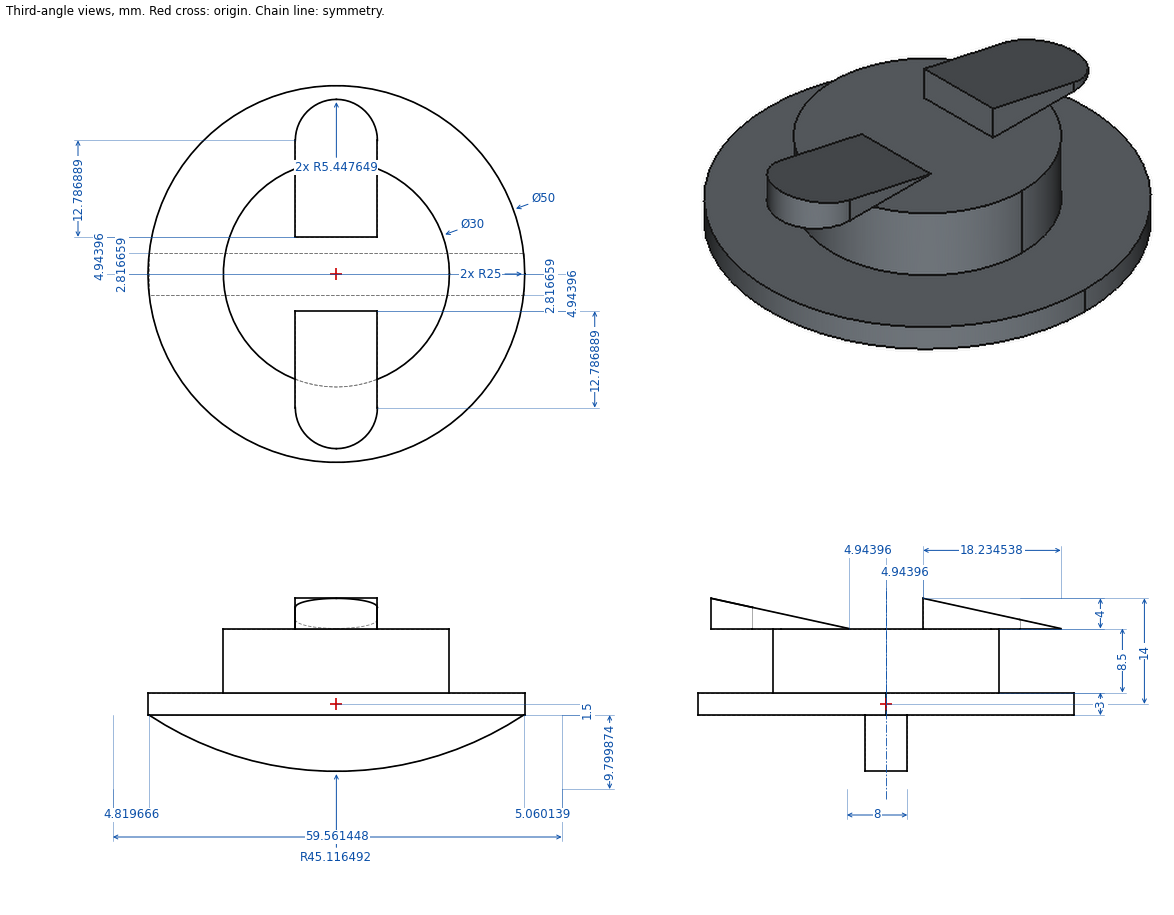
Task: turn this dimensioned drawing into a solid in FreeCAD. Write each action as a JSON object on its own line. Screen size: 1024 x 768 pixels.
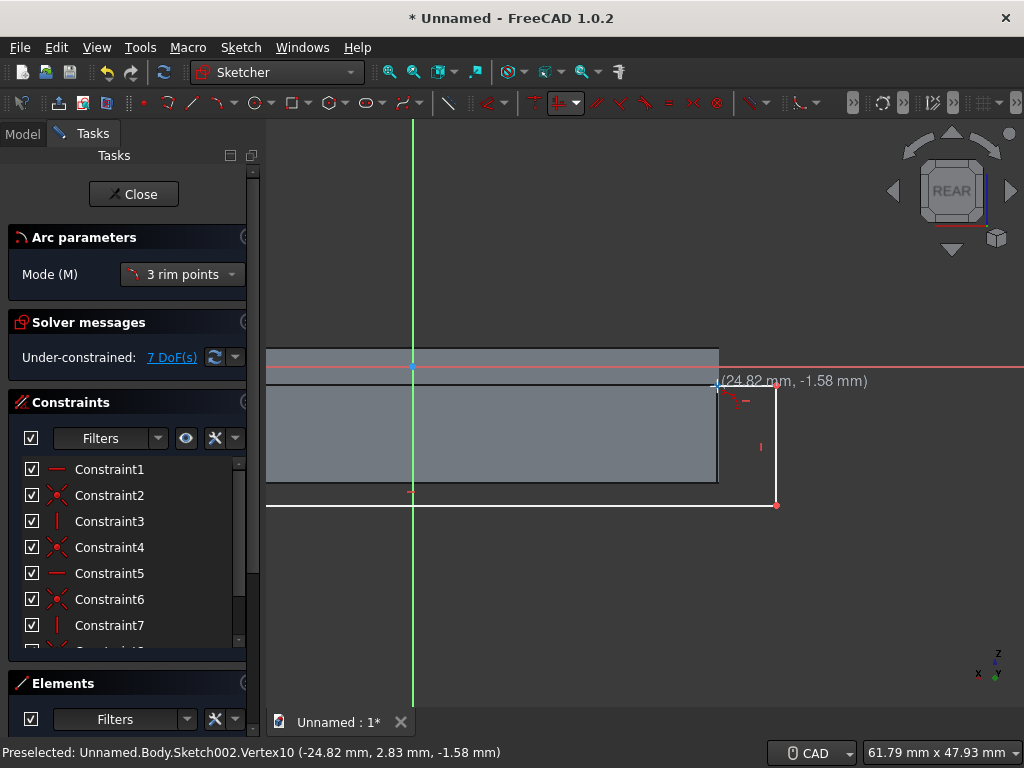
{"action": "scroll", "coordinate": [778, 385], "scroll_direction": "down", "scroll_amount": 3}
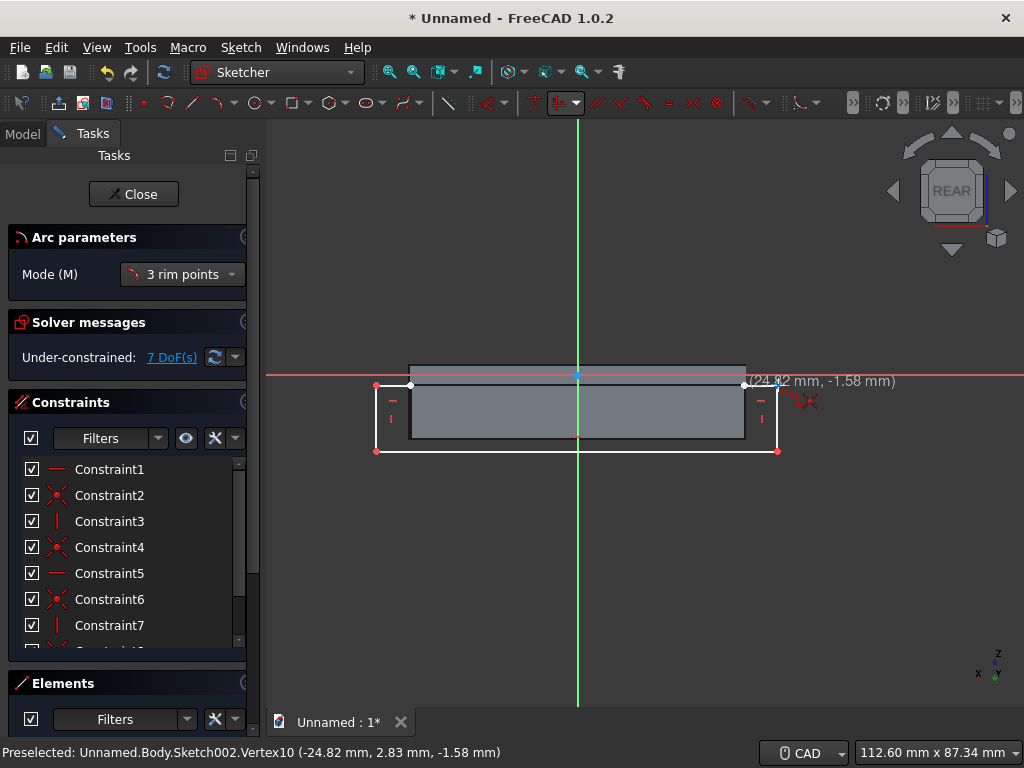
{"action": "scroll", "coordinate": [411, 385], "scroll_direction": "up", "scroll_amount": 3}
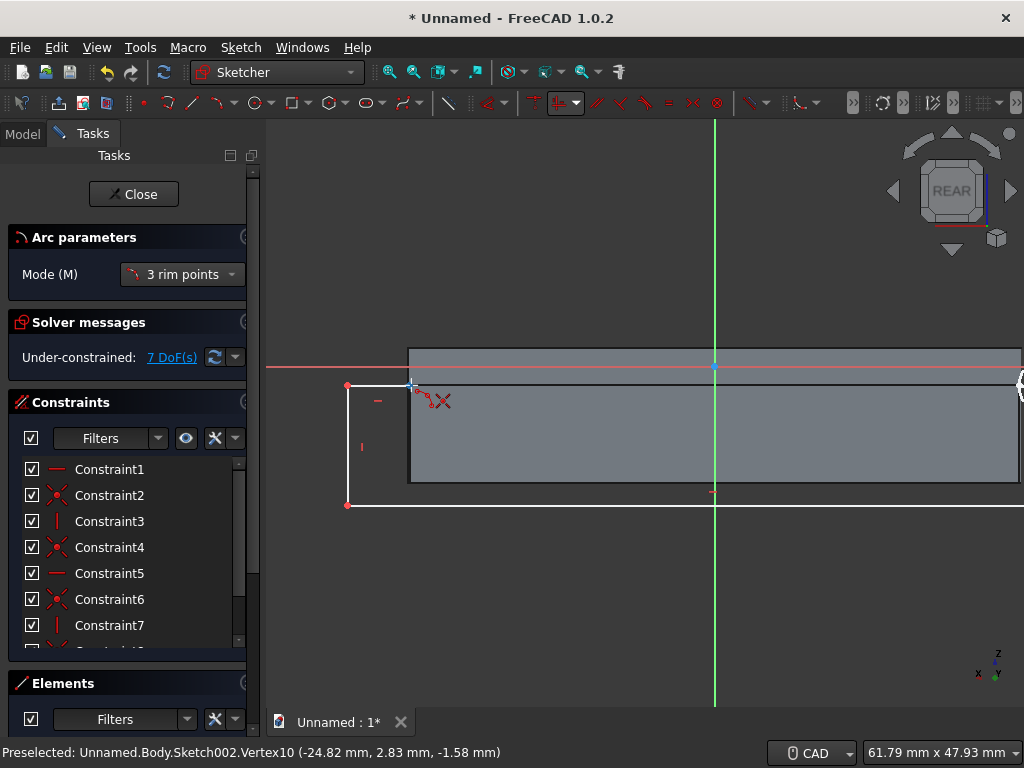
{"action": "left_click", "coordinate": [410, 386]}
{"action": "left_click", "coordinate": [650, 473]}
{"action": "key", "text": "Escape"}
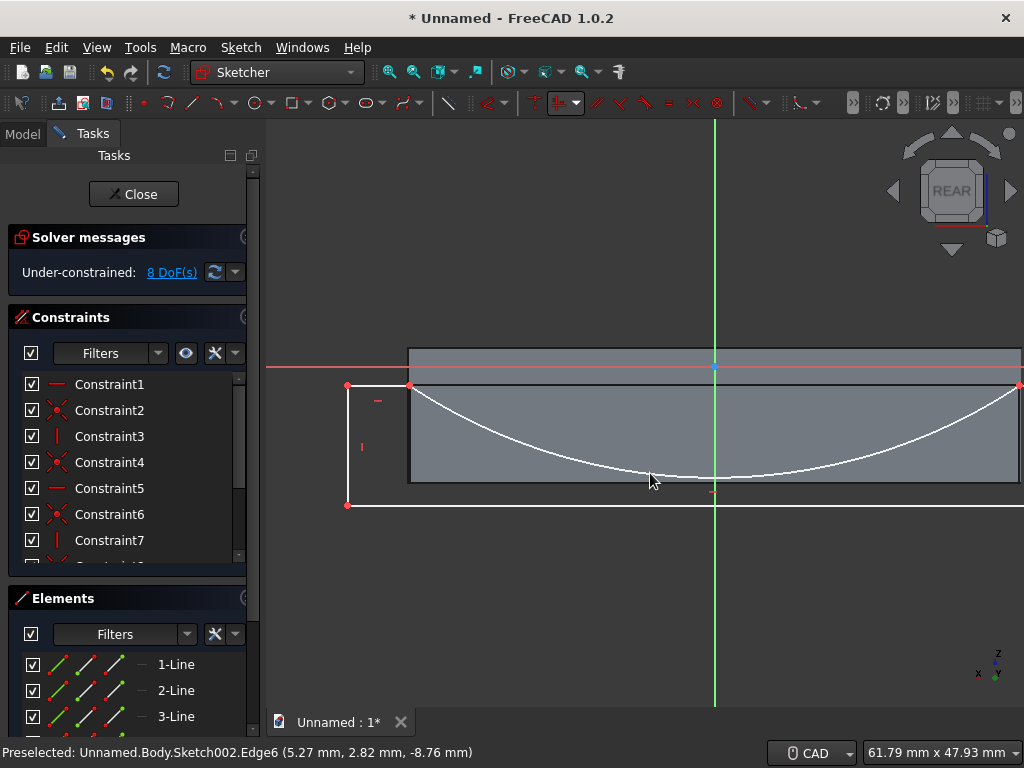
{"action": "scroll", "coordinate": [410, 385], "scroll_direction": "down", "scroll_amount": 3}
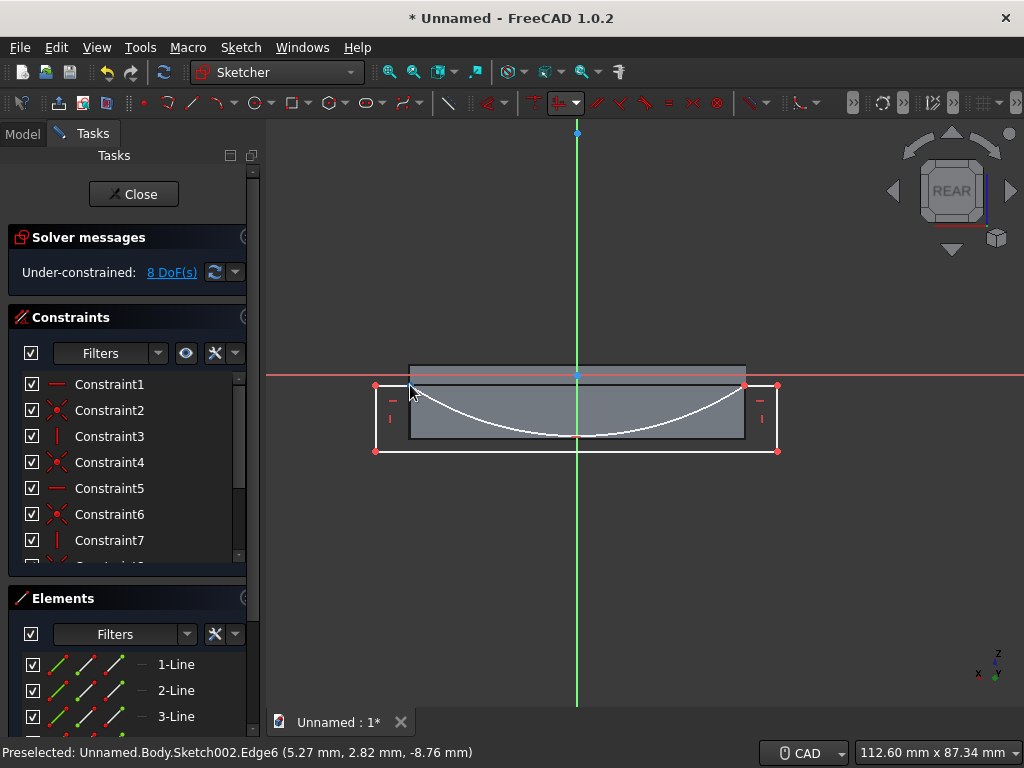
{"action": "scroll", "coordinate": [576, 679], "scroll_direction": "down", "scroll_amount": 1}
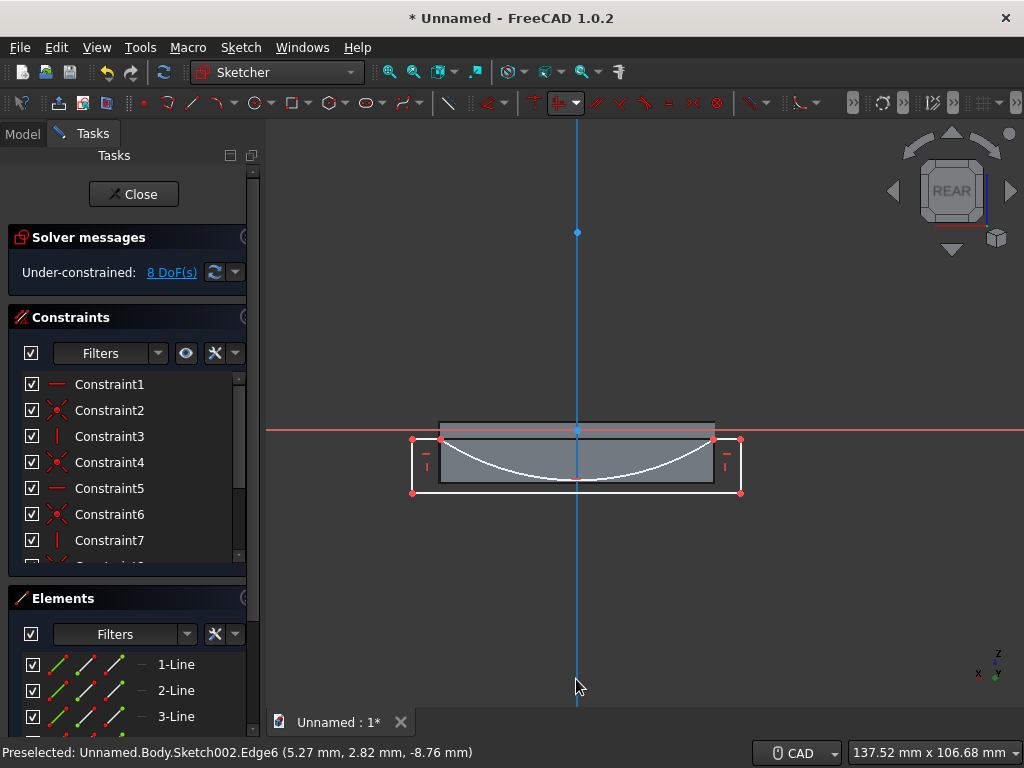
{"action": "left_click", "coordinate": [577, 233]}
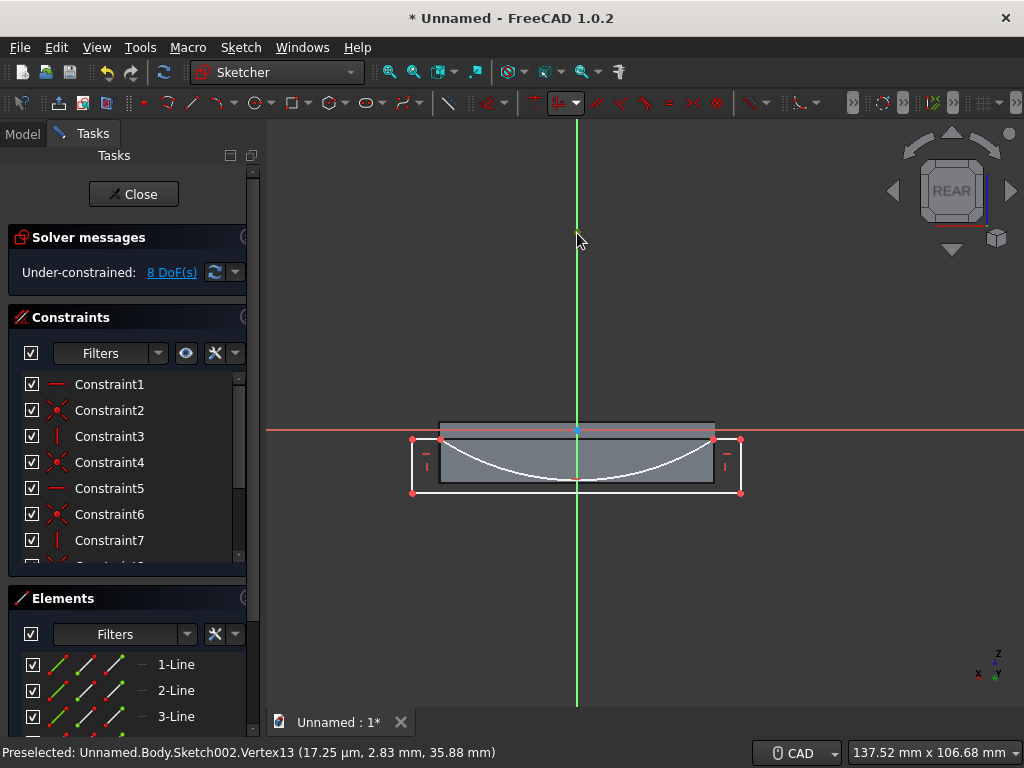
{"action": "left_click", "coordinate": [577, 641]}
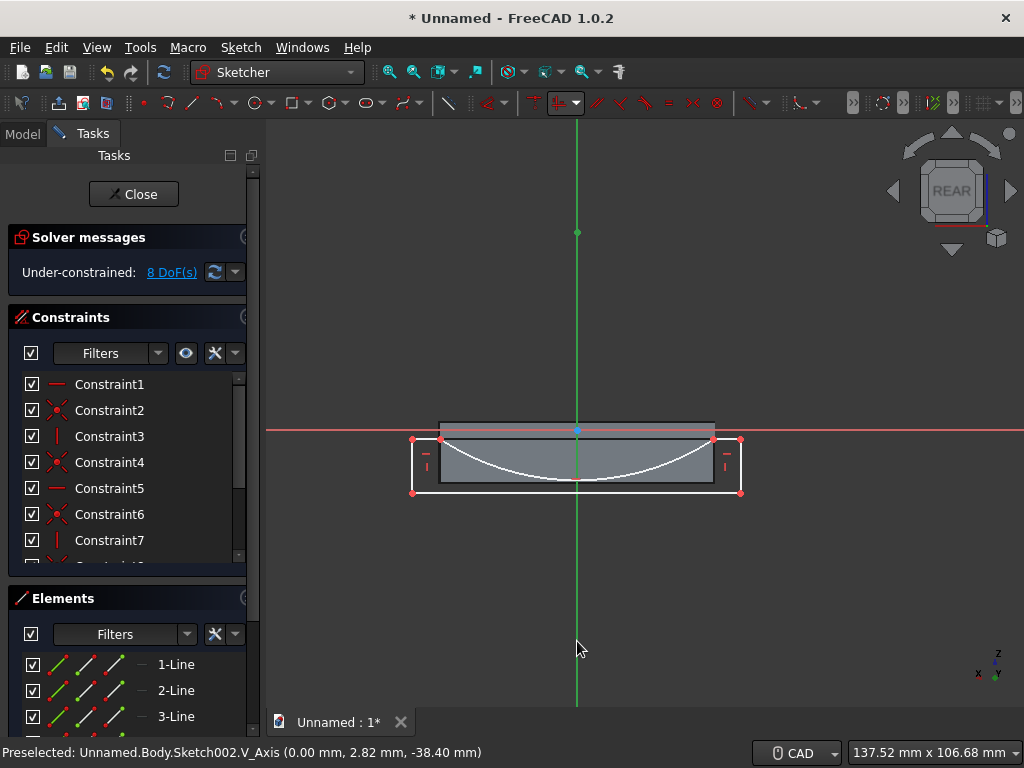
{"action": "left_click", "coordinate": [534, 104]}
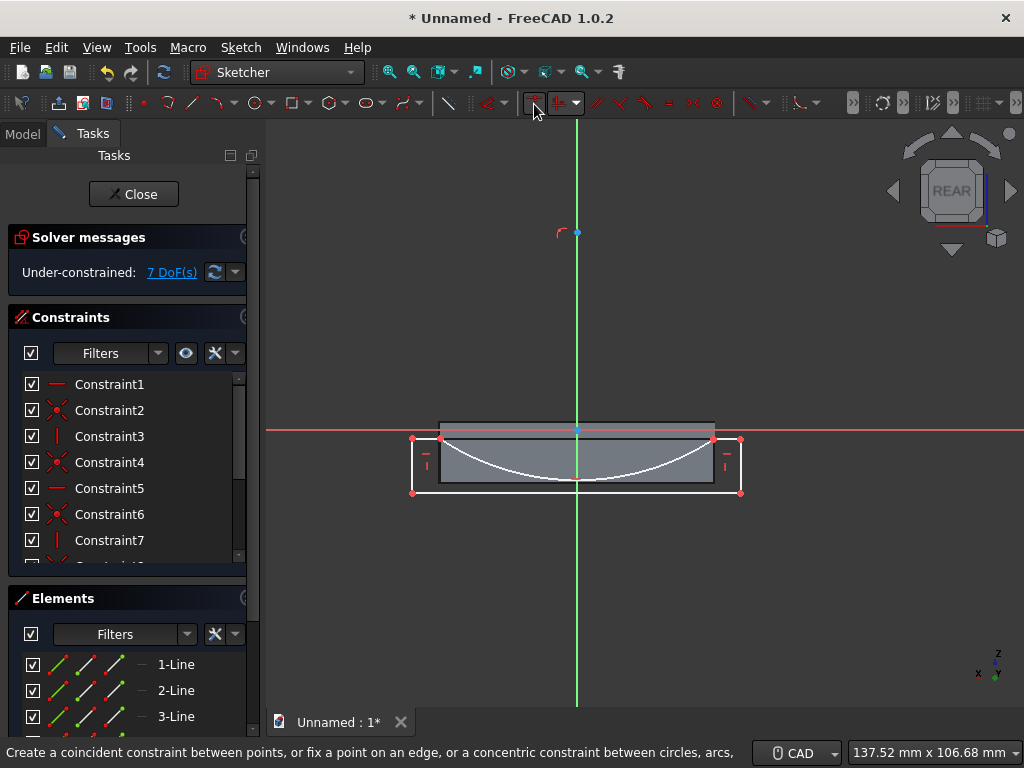
{"action": "left_click", "coordinate": [488, 104]}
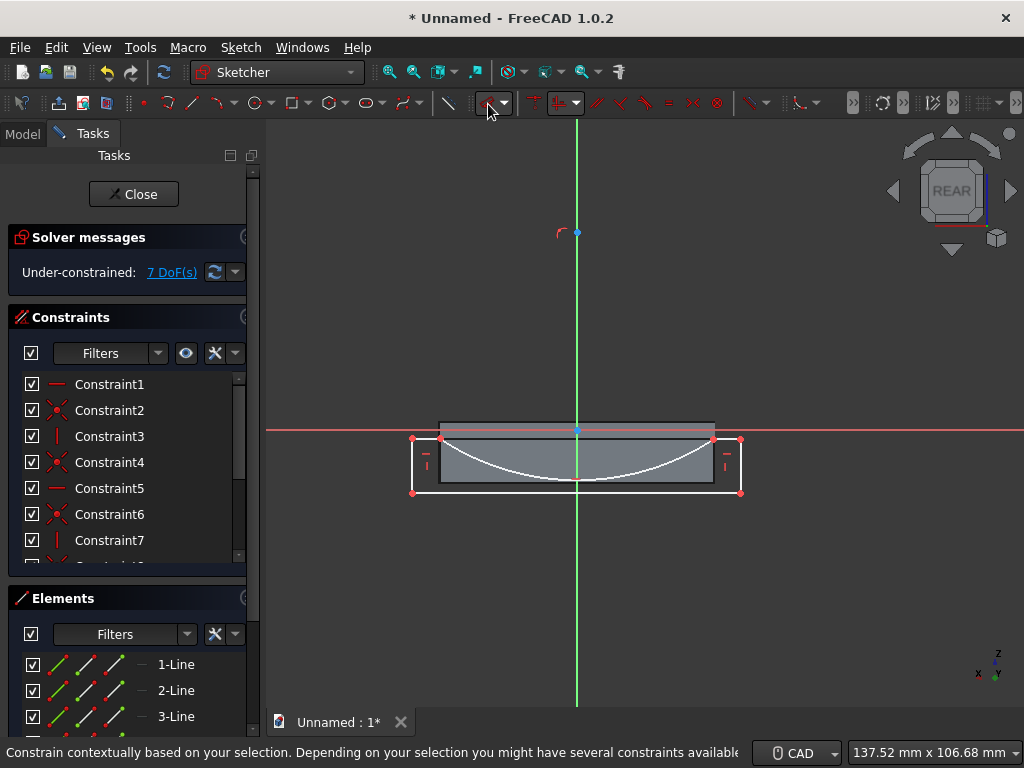
{"action": "left_click", "coordinate": [520, 473]}
{"action": "left_click", "coordinate": [314, 325]}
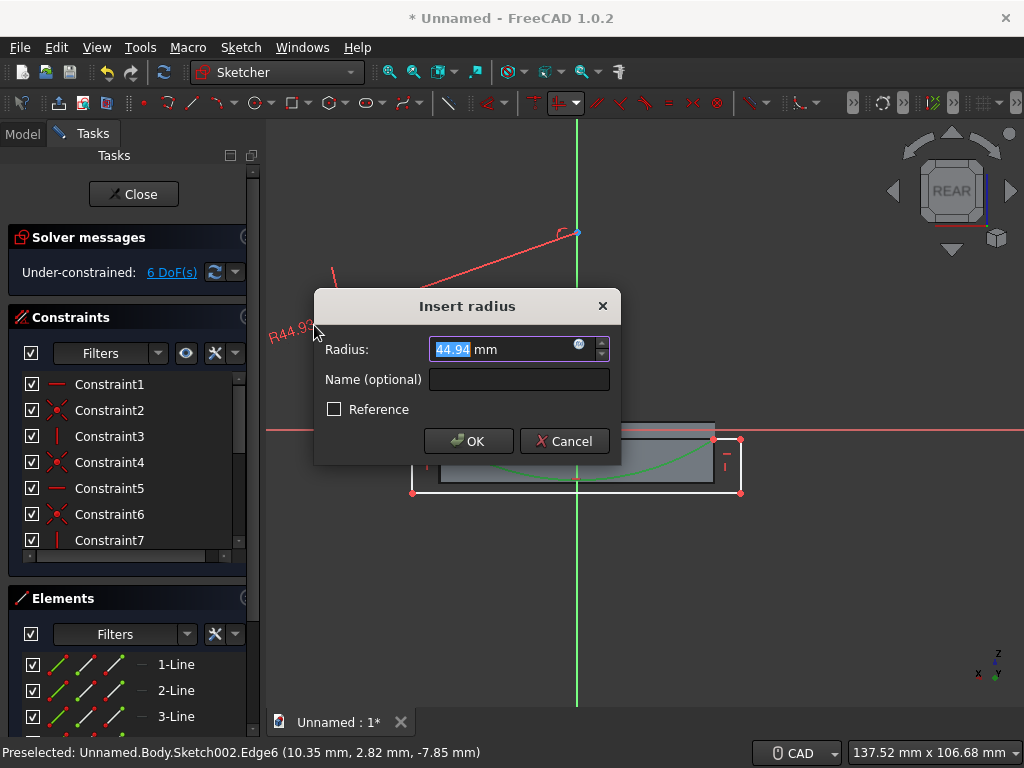
{"action": "type", "text": "45.116492"}
{"action": "key", "text": "Return"}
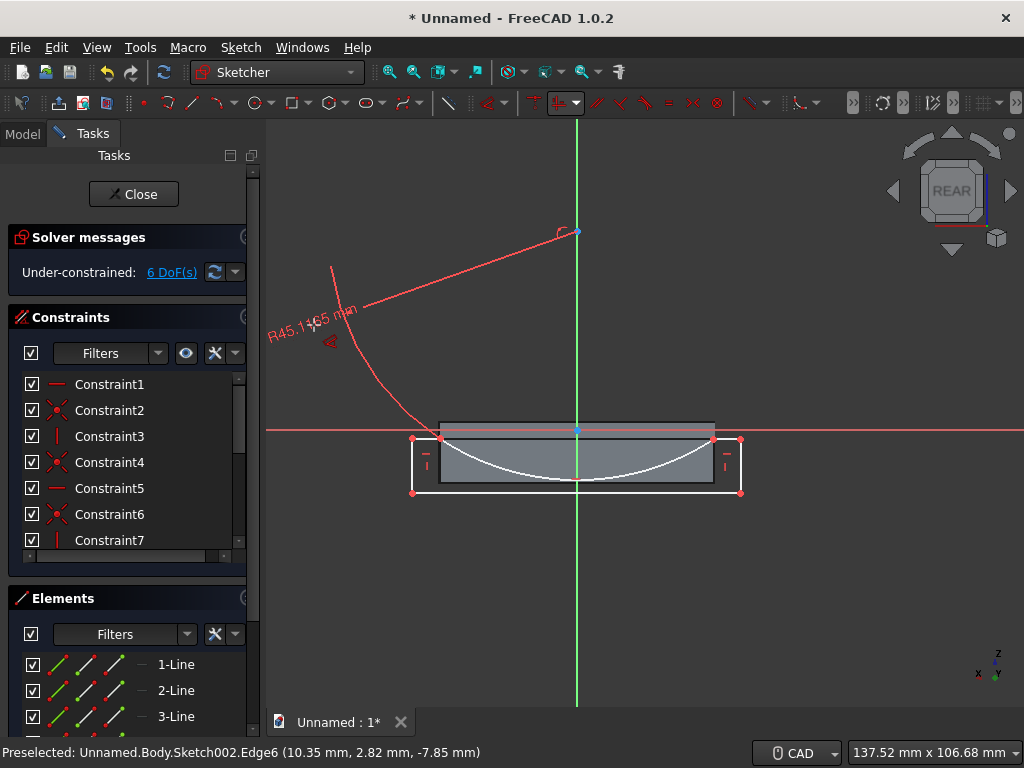
{"action": "scroll", "coordinate": [440, 439], "scroll_direction": "up", "scroll_amount": 8}